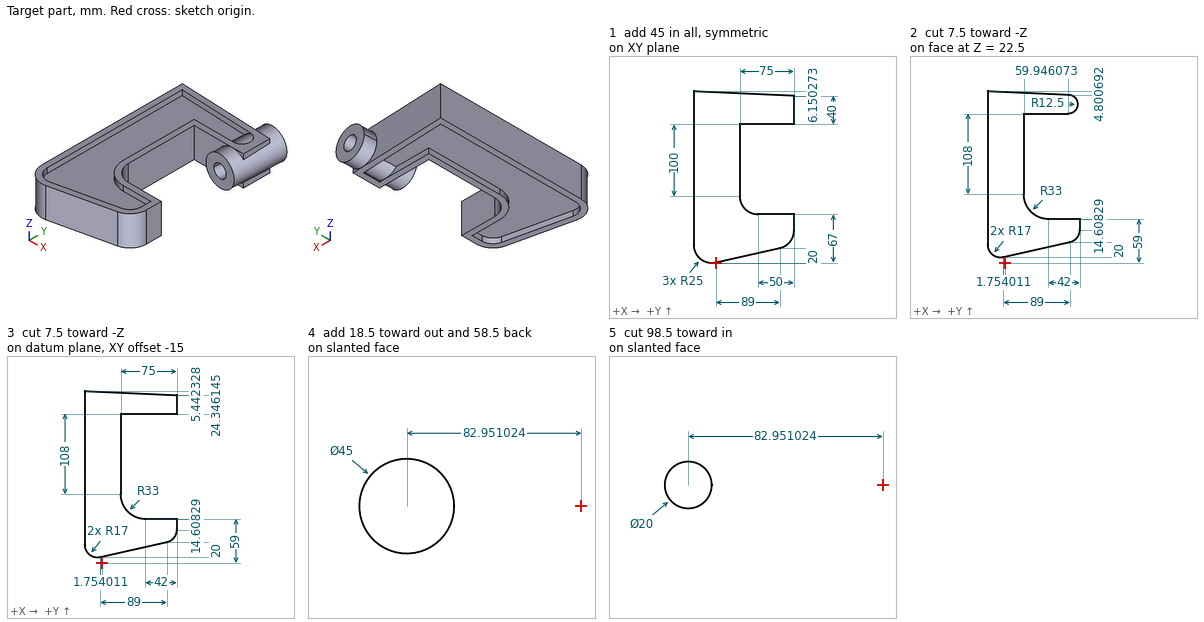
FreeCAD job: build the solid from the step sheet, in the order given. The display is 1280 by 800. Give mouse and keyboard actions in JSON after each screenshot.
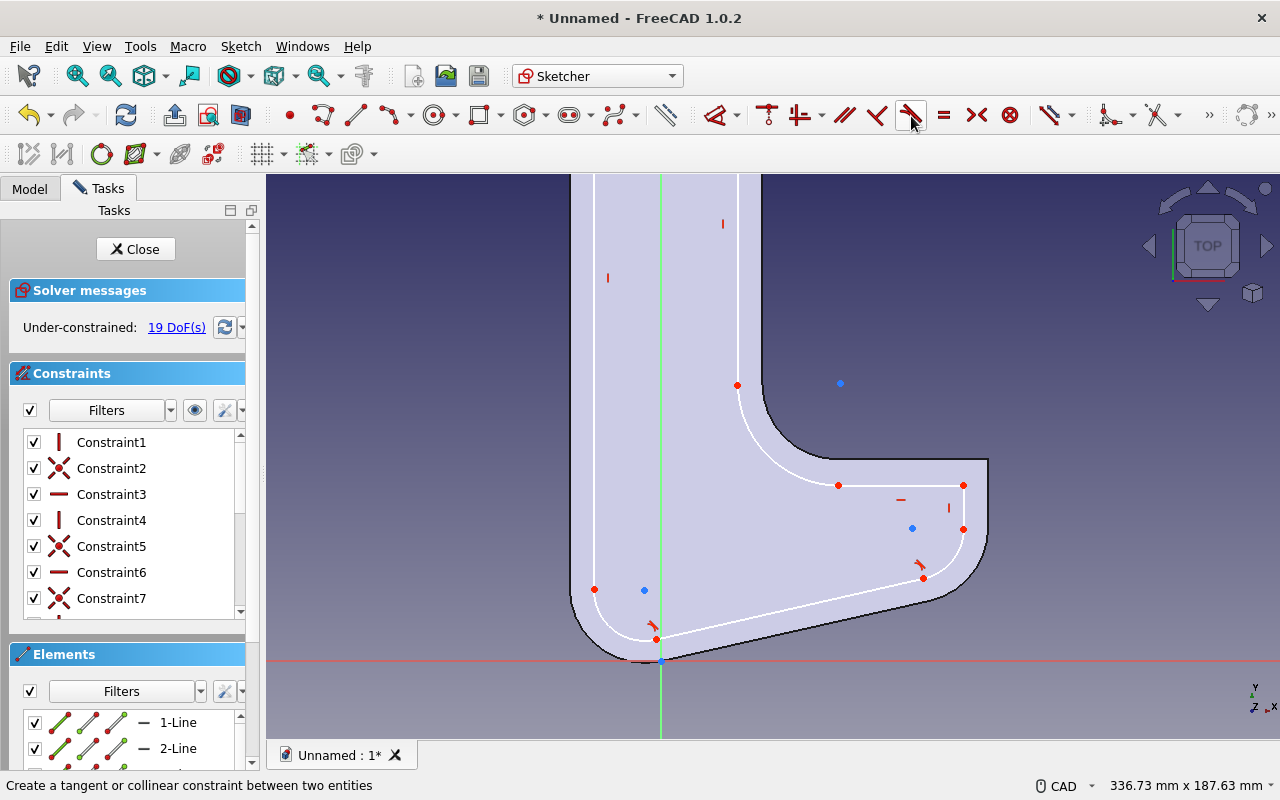
{"action": "left_click", "coordinate": [964, 516]}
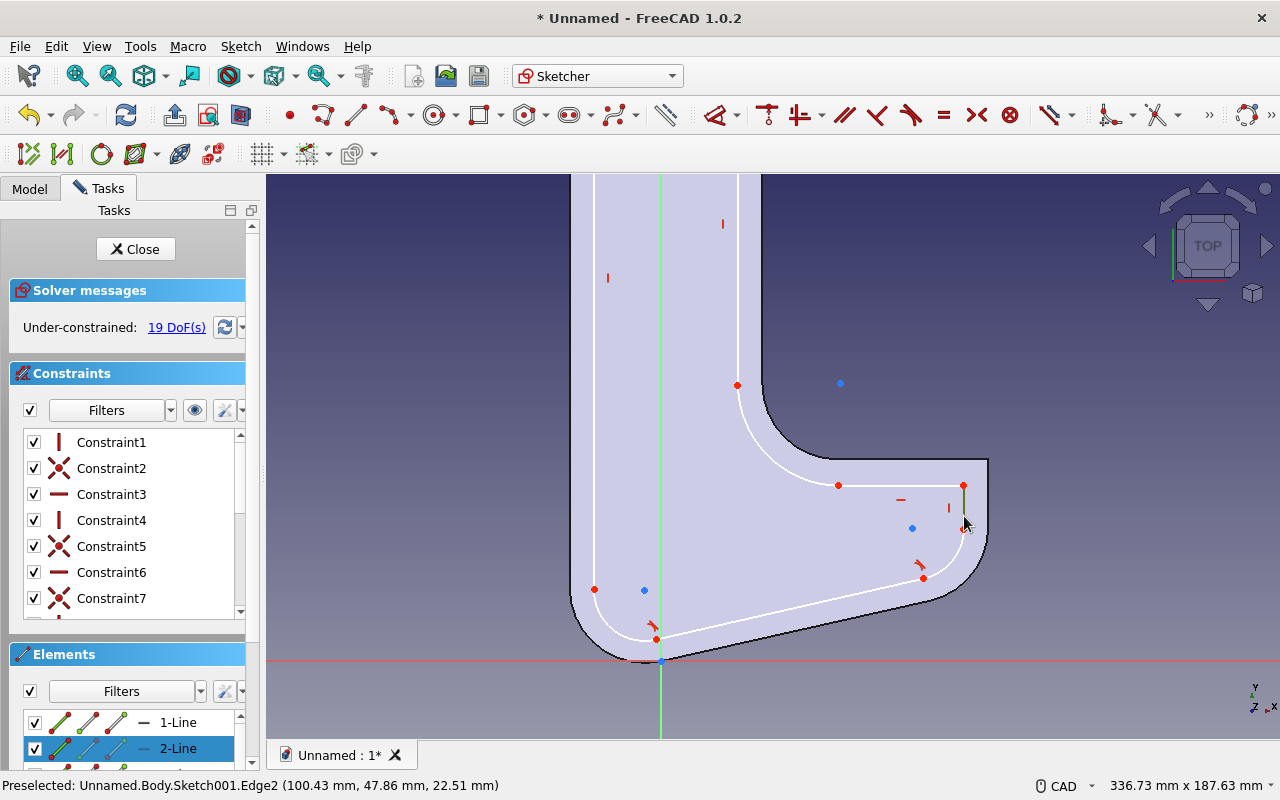
{"action": "left_click", "coordinate": [942, 570]}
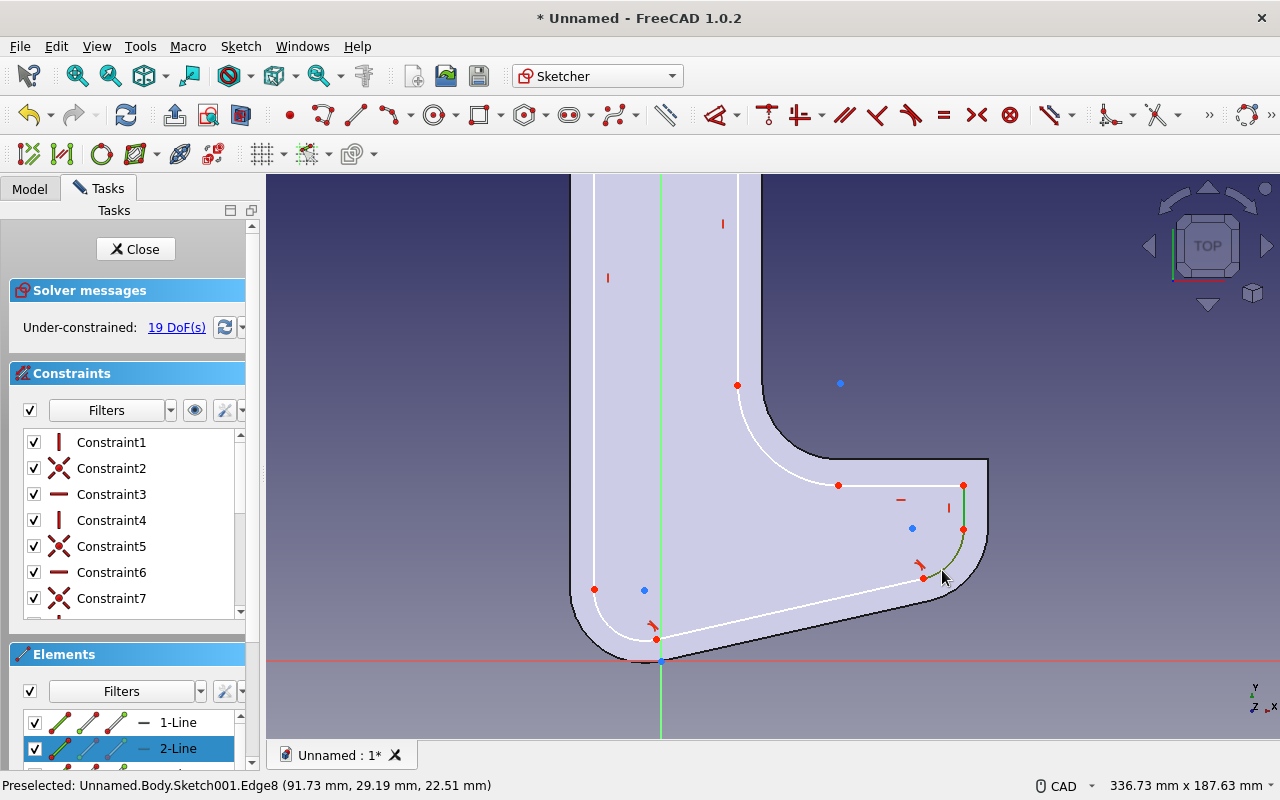
{"action": "key", "text": "t"}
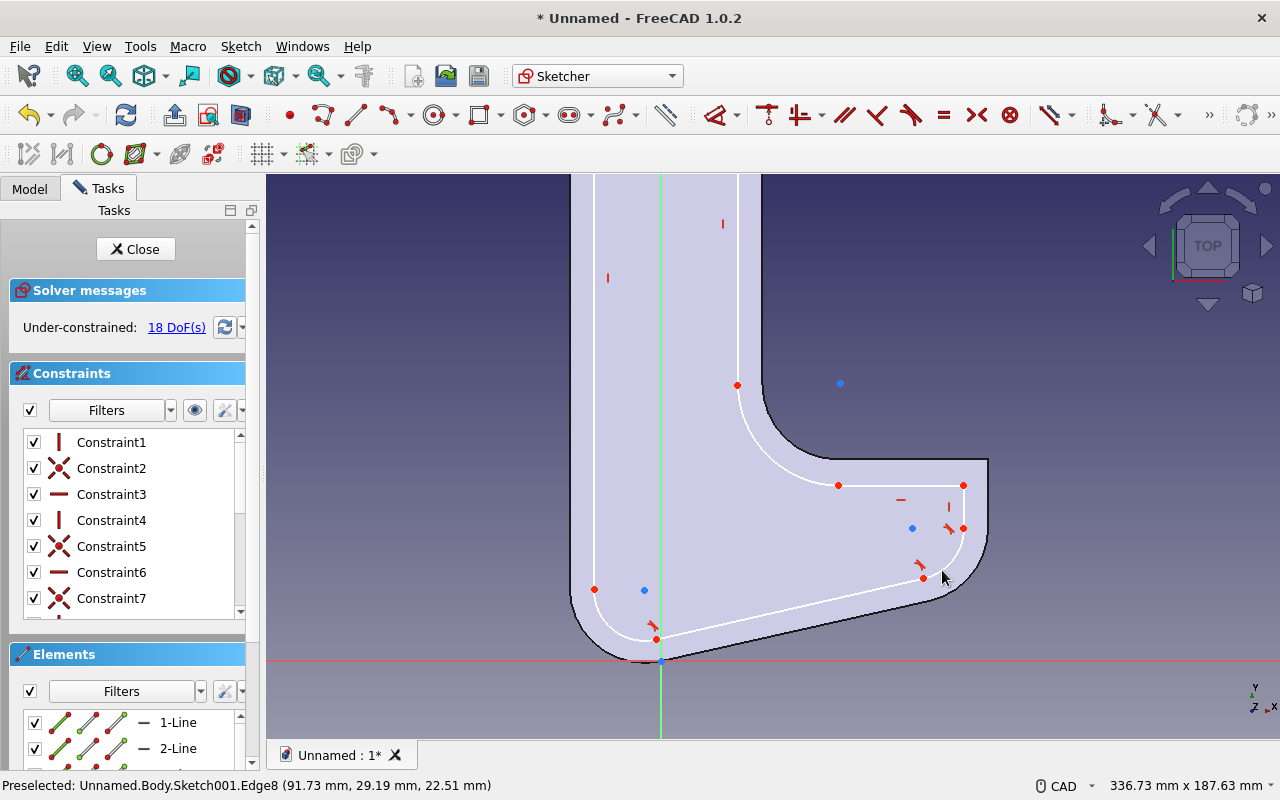
{"action": "left_click", "coordinate": [926, 486]}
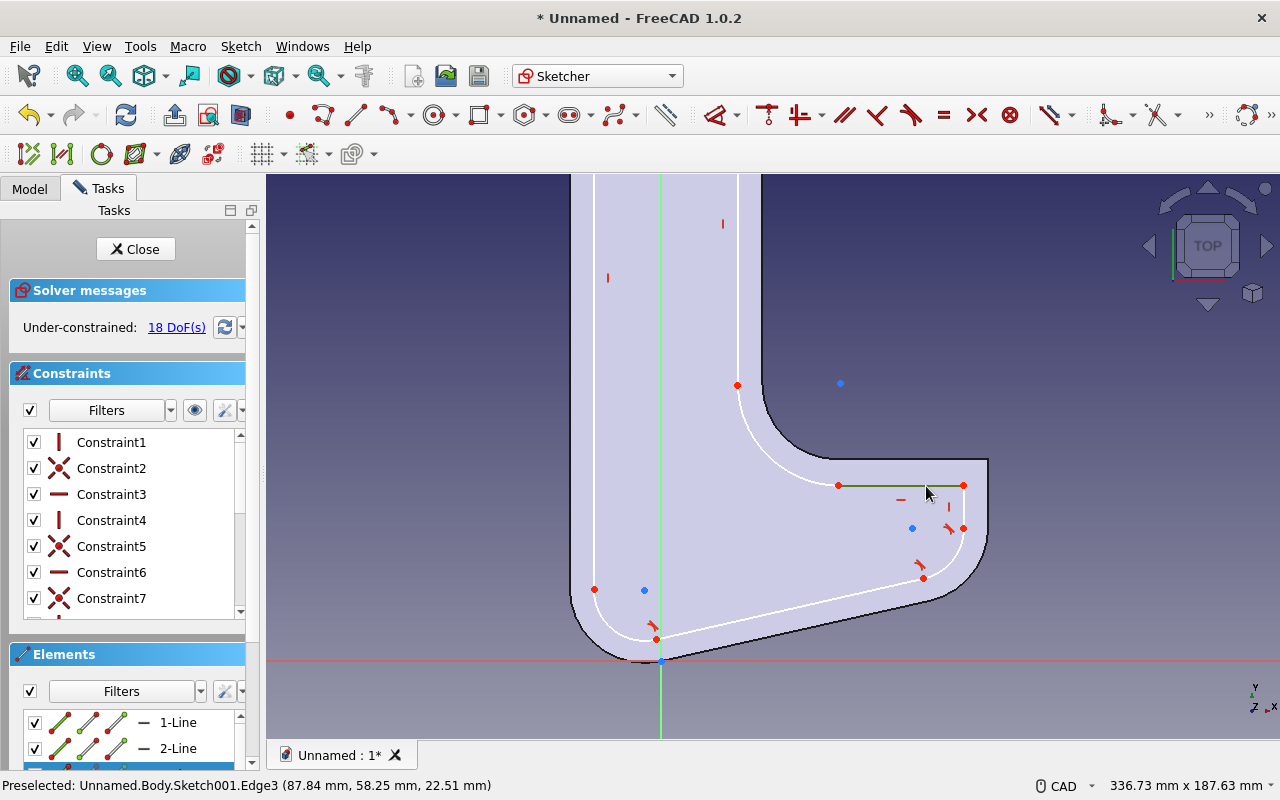
{"action": "left_click", "coordinate": [750, 431]}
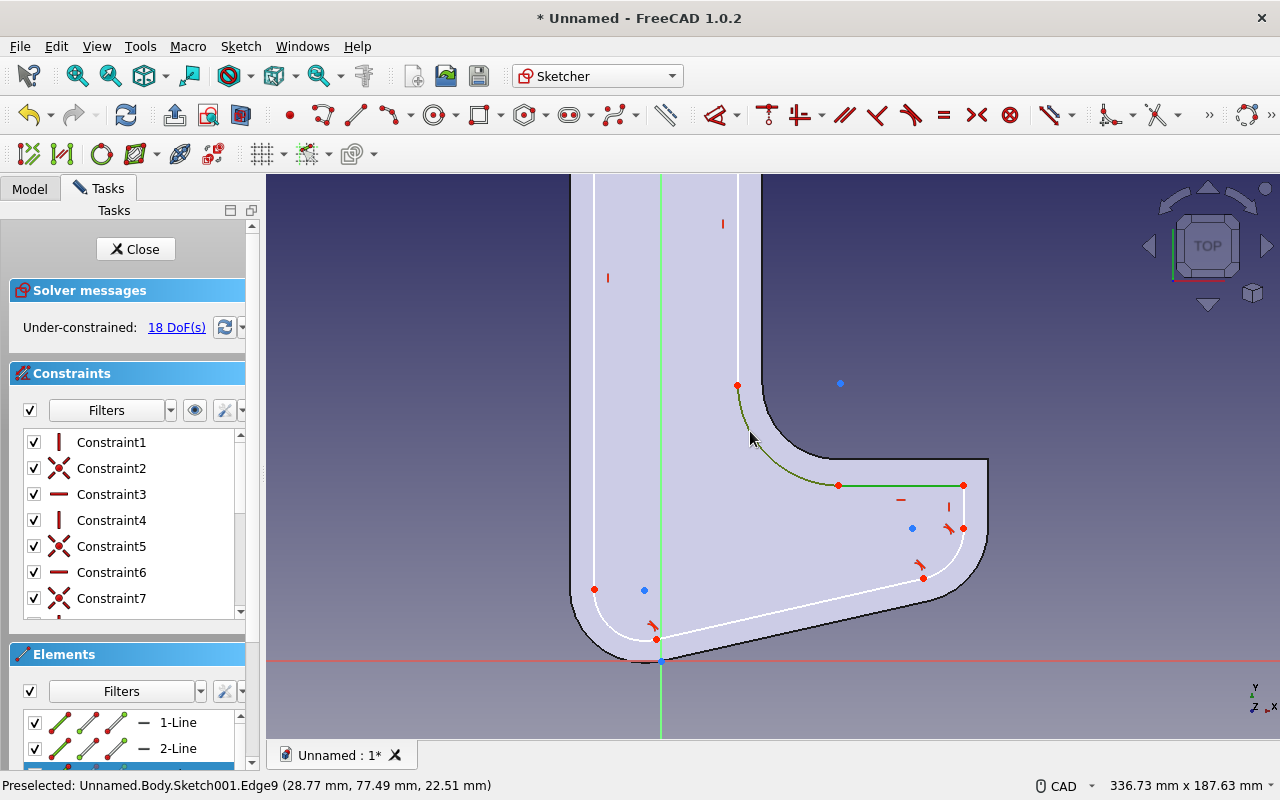
{"action": "left_click", "coordinate": [911, 116]}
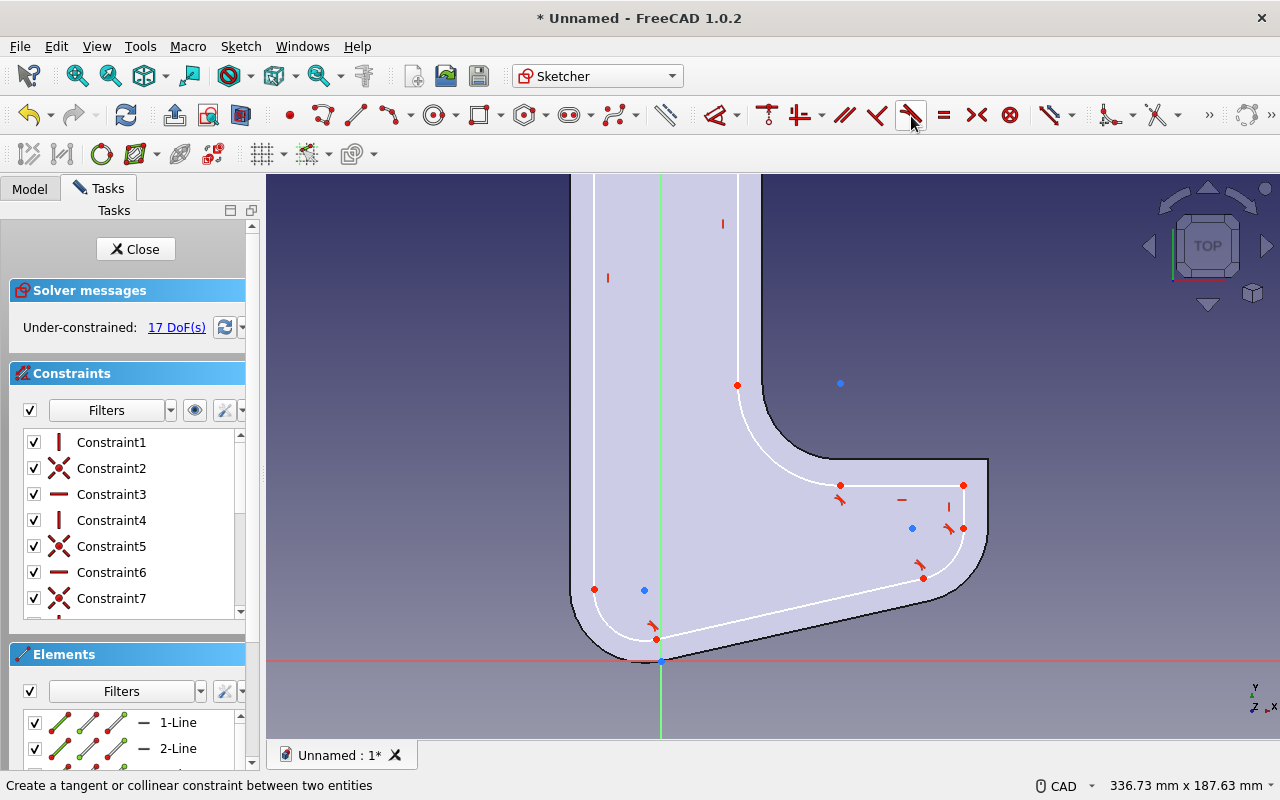
{"action": "left_click", "coordinate": [738, 288]}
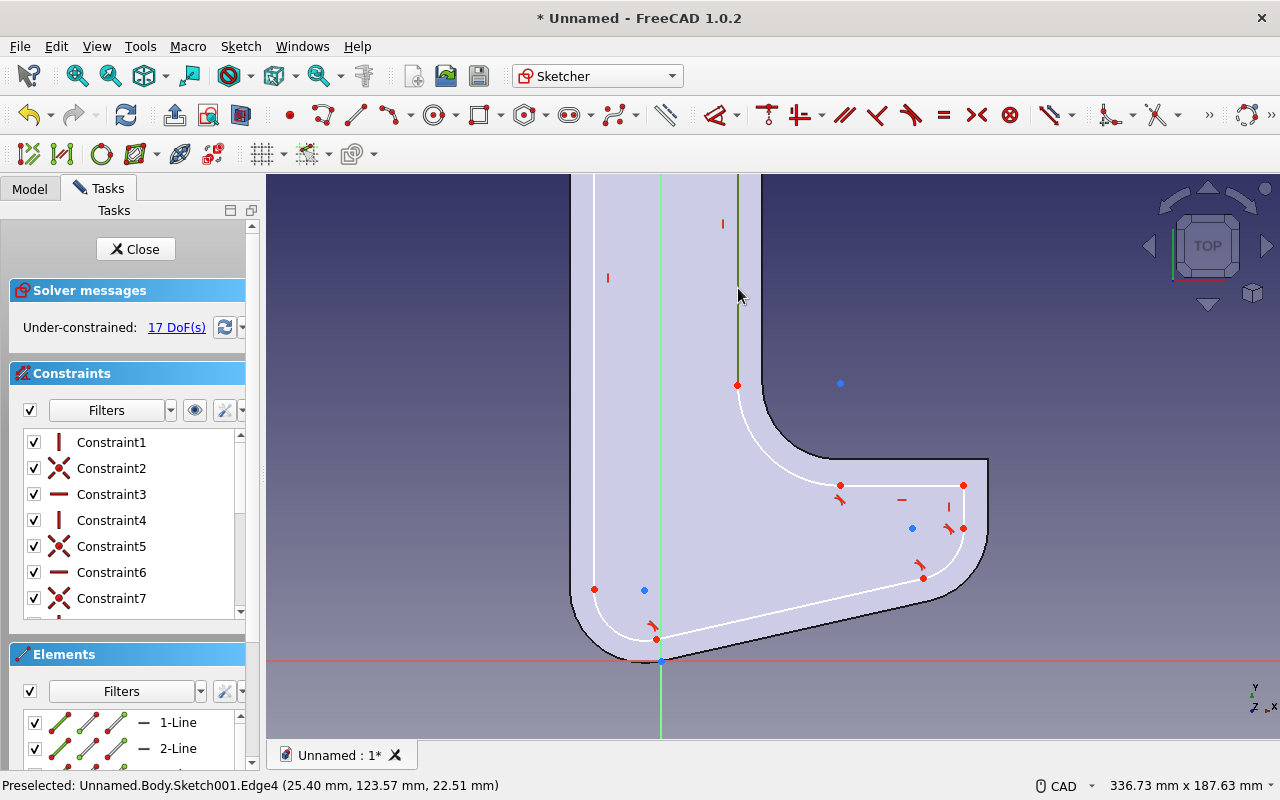
{"action": "left_click", "coordinate": [750, 431]}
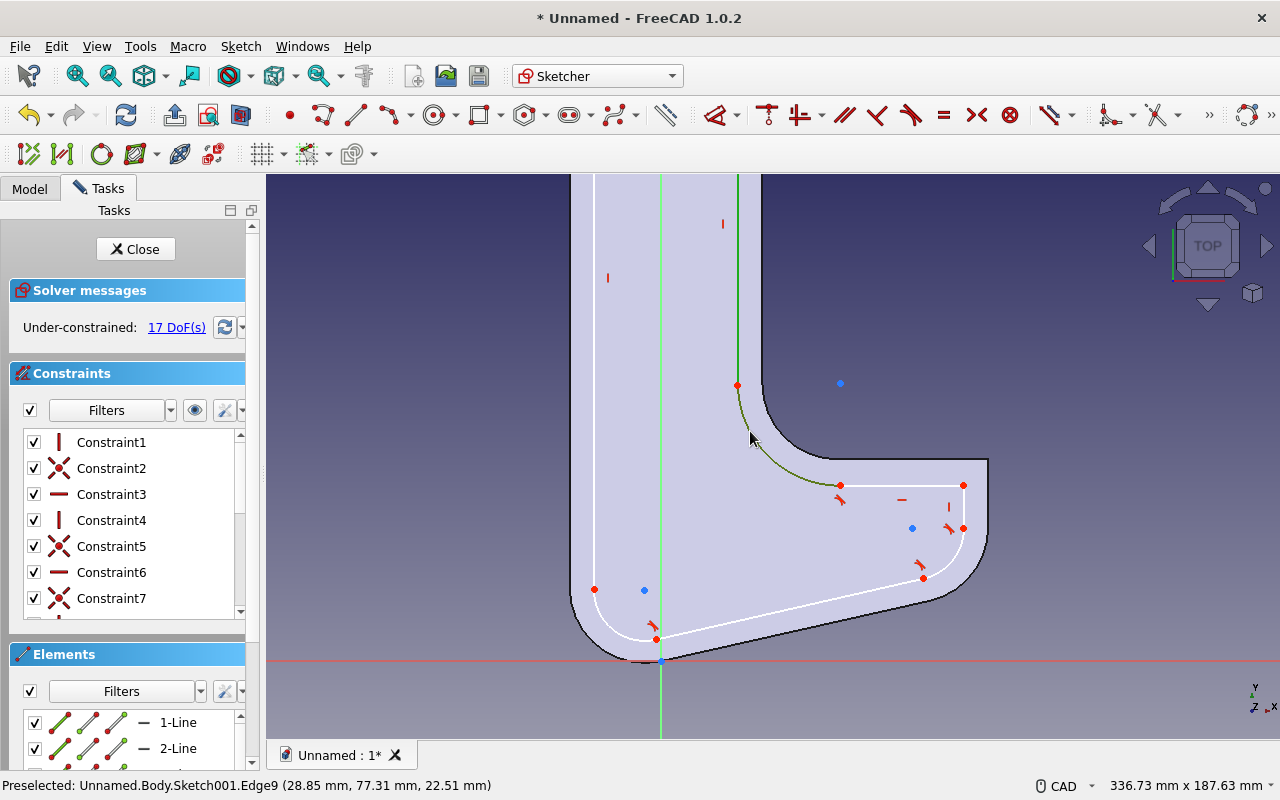
{"action": "left_click", "coordinate": [911, 116]}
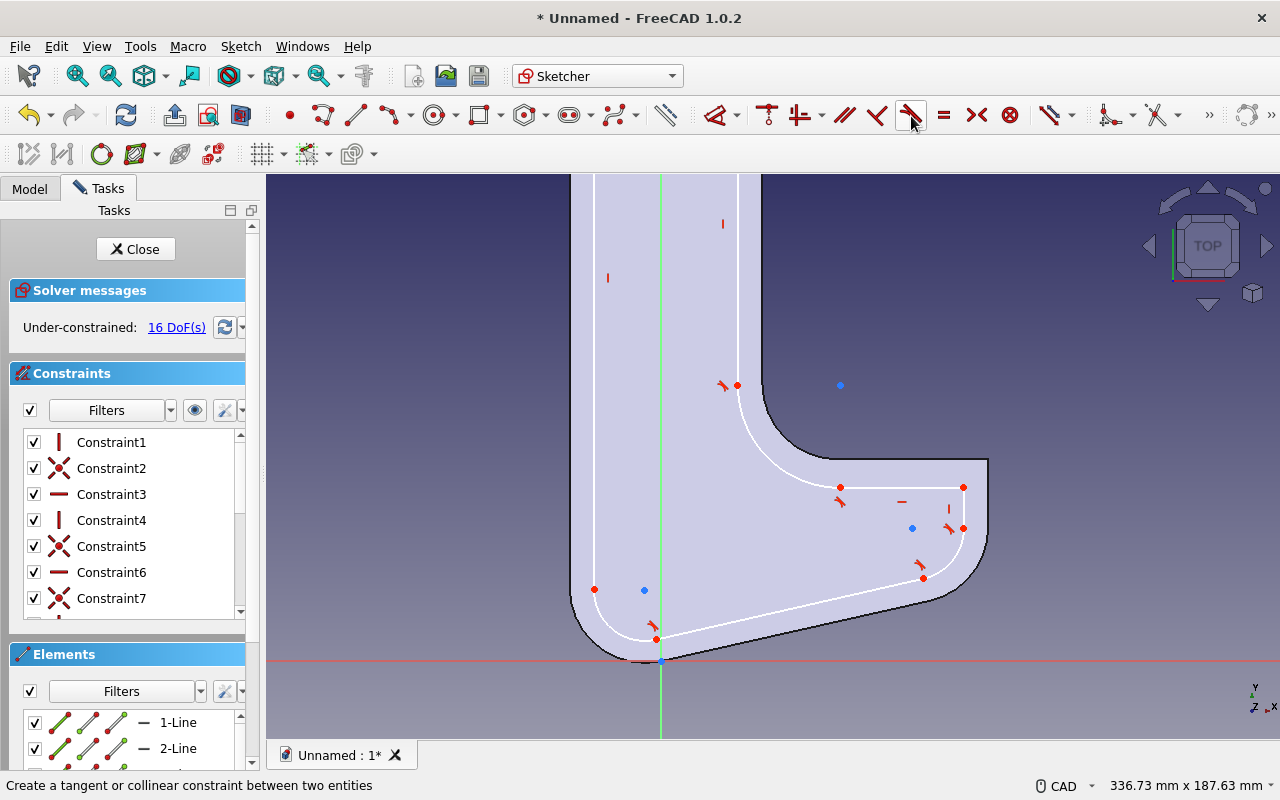
{"action": "scroll", "coordinate": [614, 628], "scroll_direction": "down", "scroll_amount": 3}